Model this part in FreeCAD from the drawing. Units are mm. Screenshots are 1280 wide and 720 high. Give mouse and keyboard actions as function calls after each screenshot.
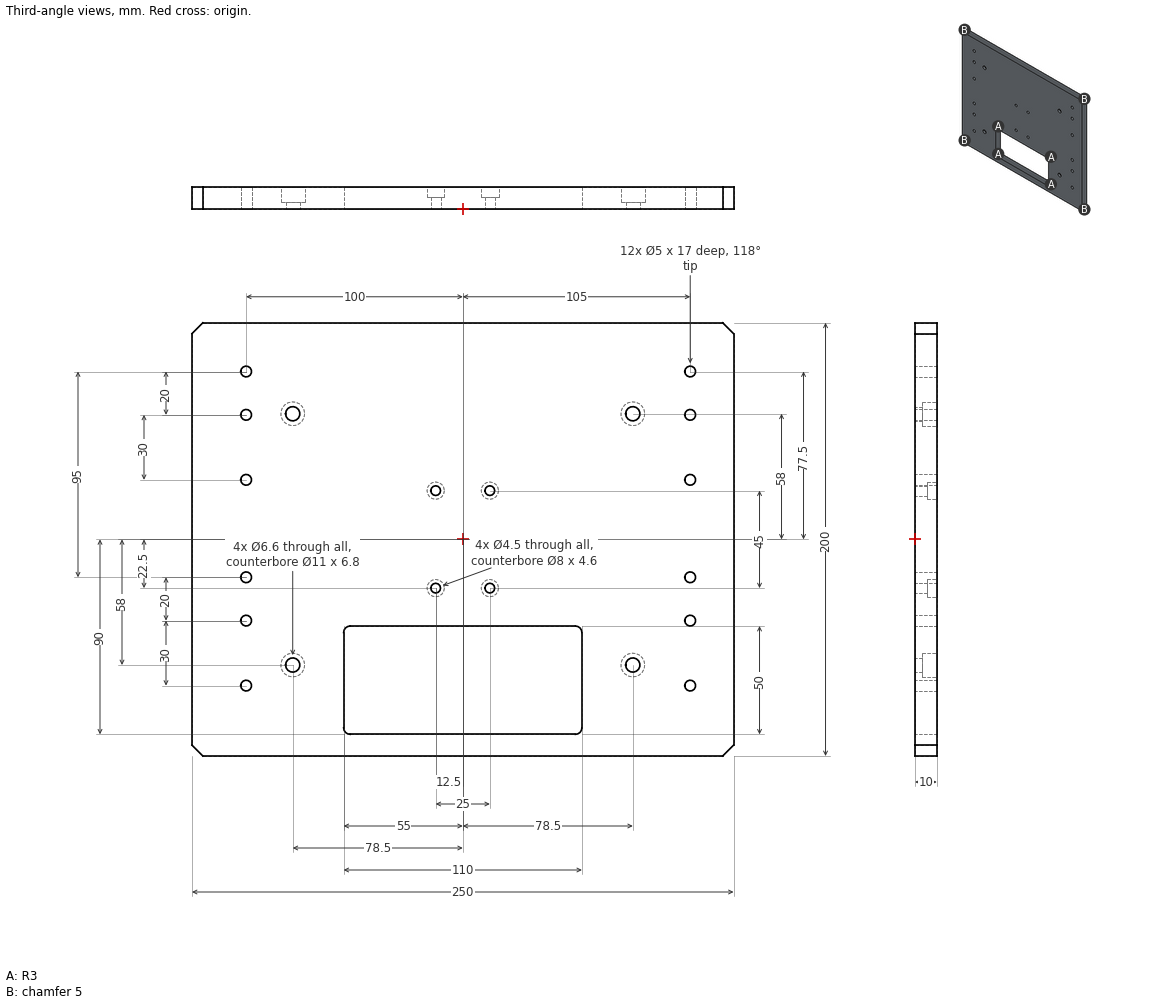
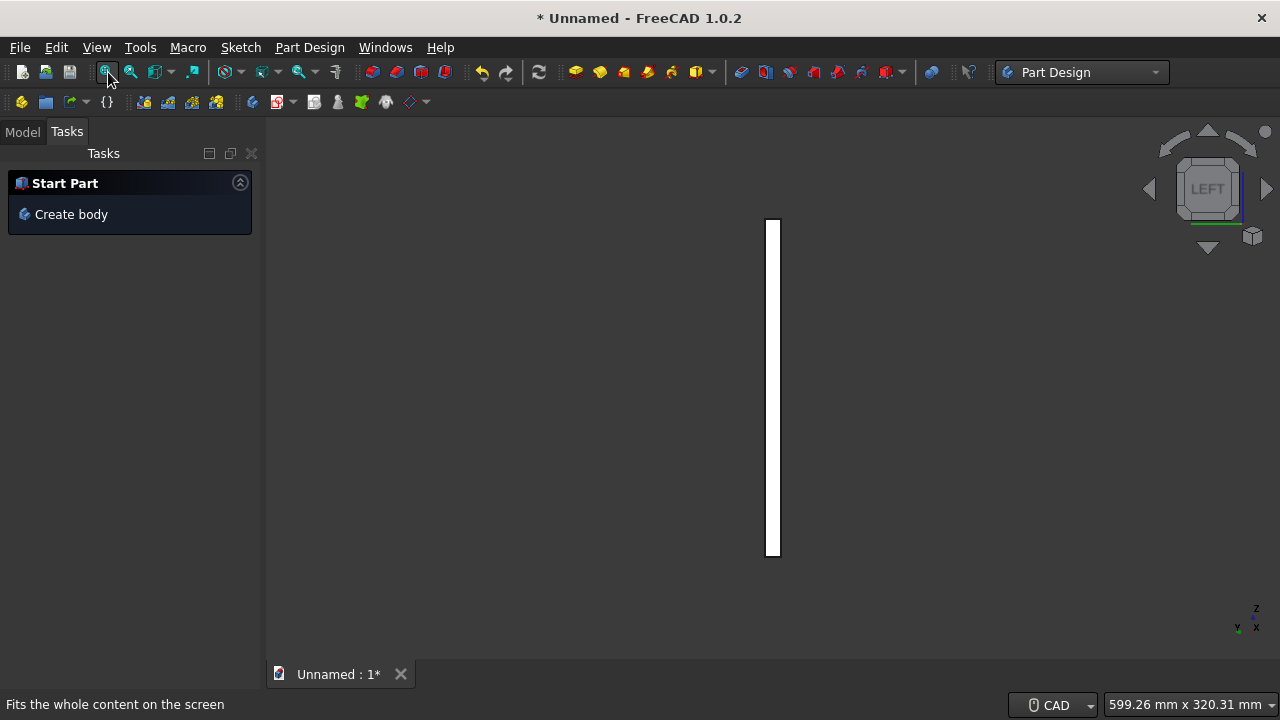
scroll(773, 455, up, 5)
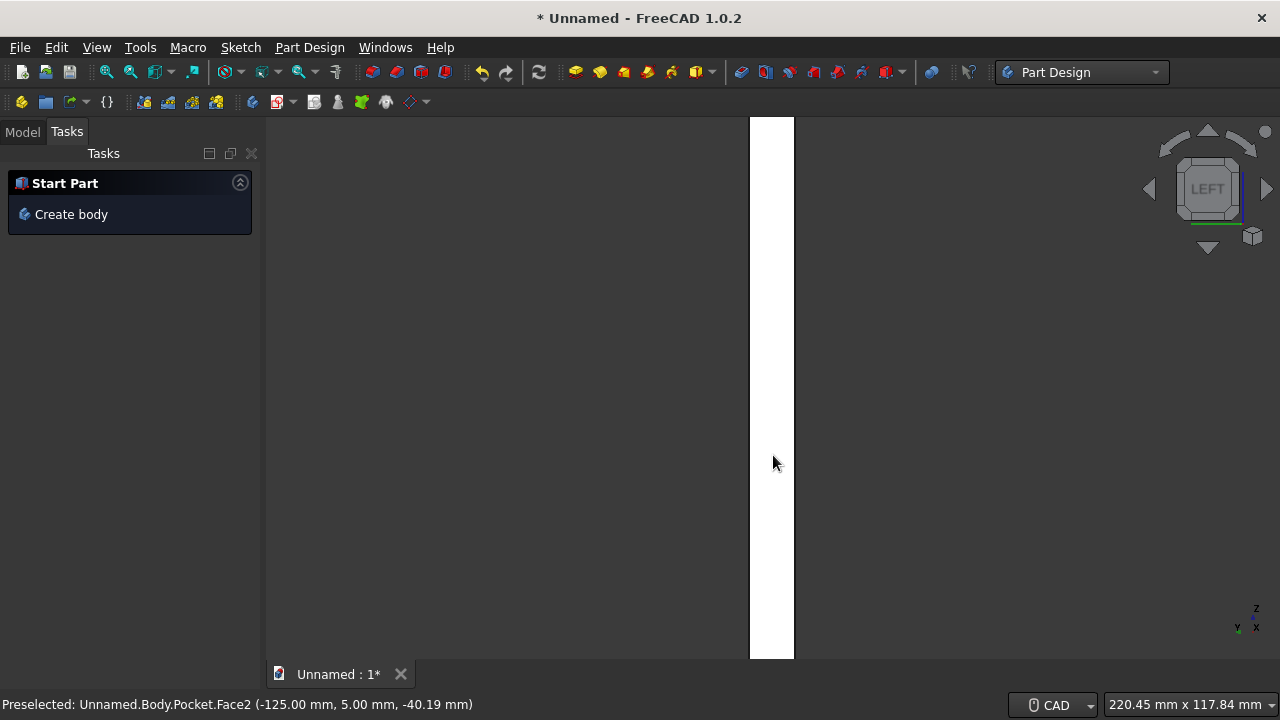
click(108, 72)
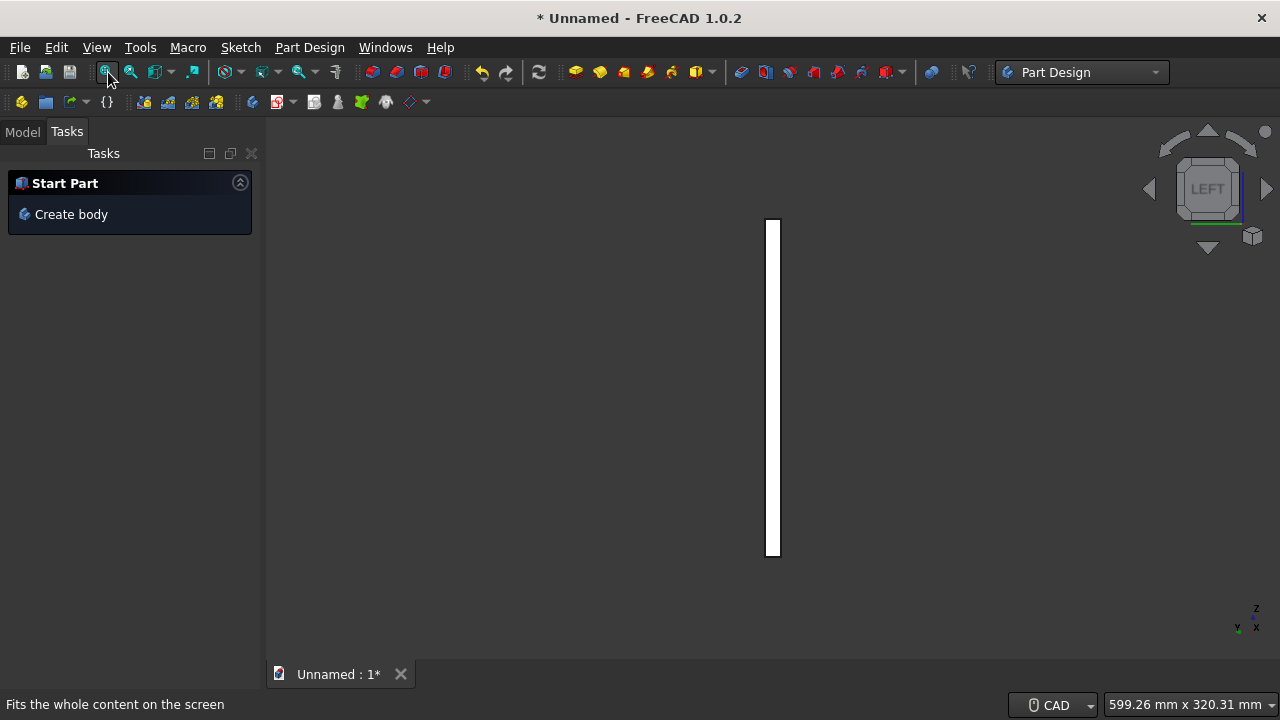
key(v)
key(3)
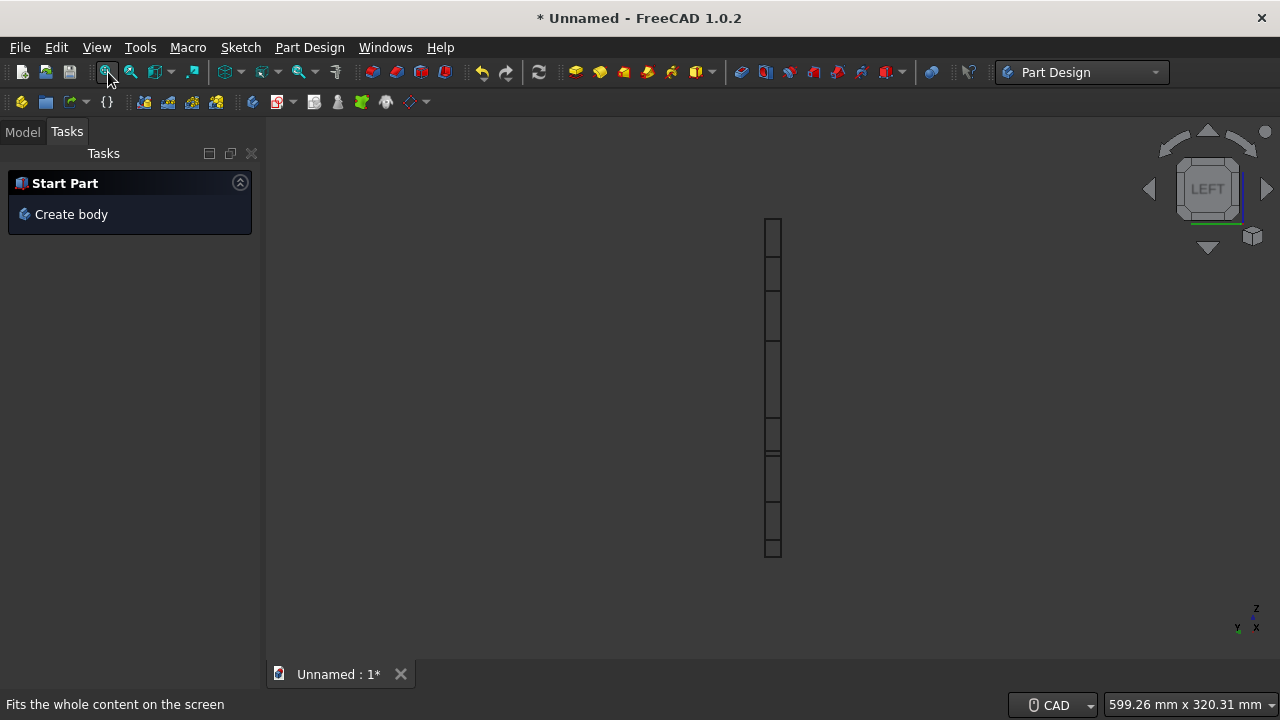
key(0)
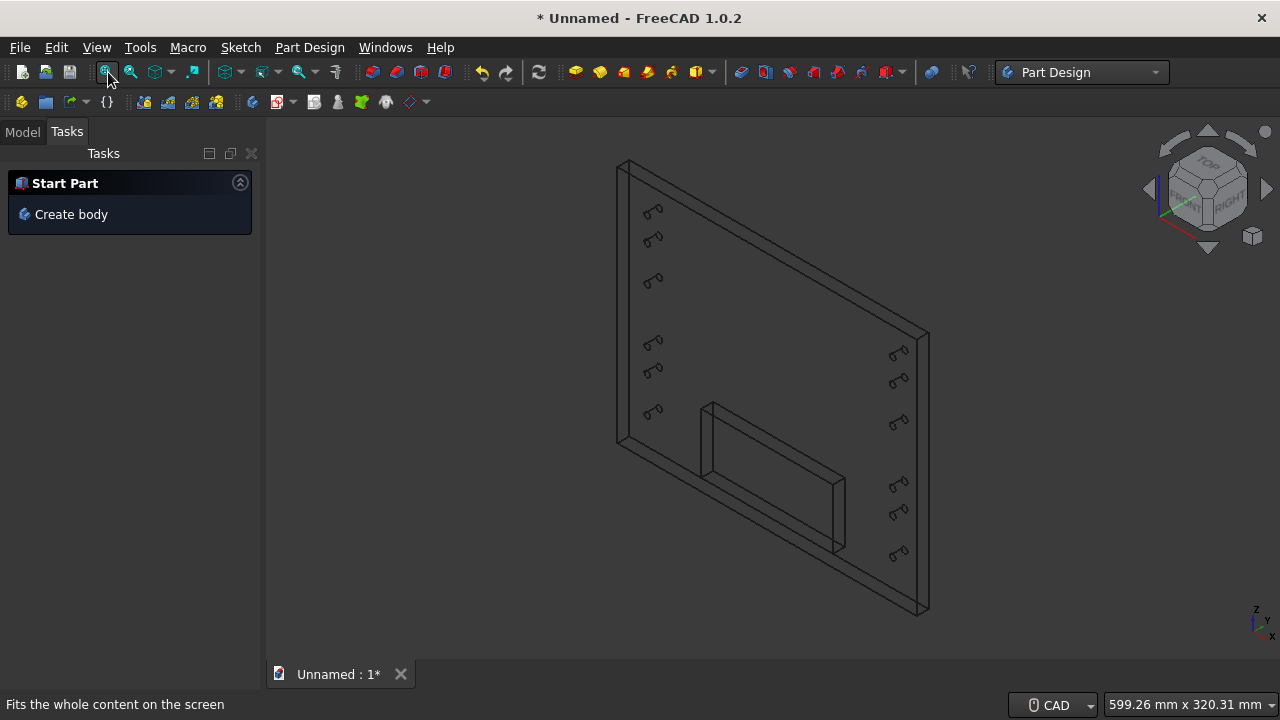
click(708, 404)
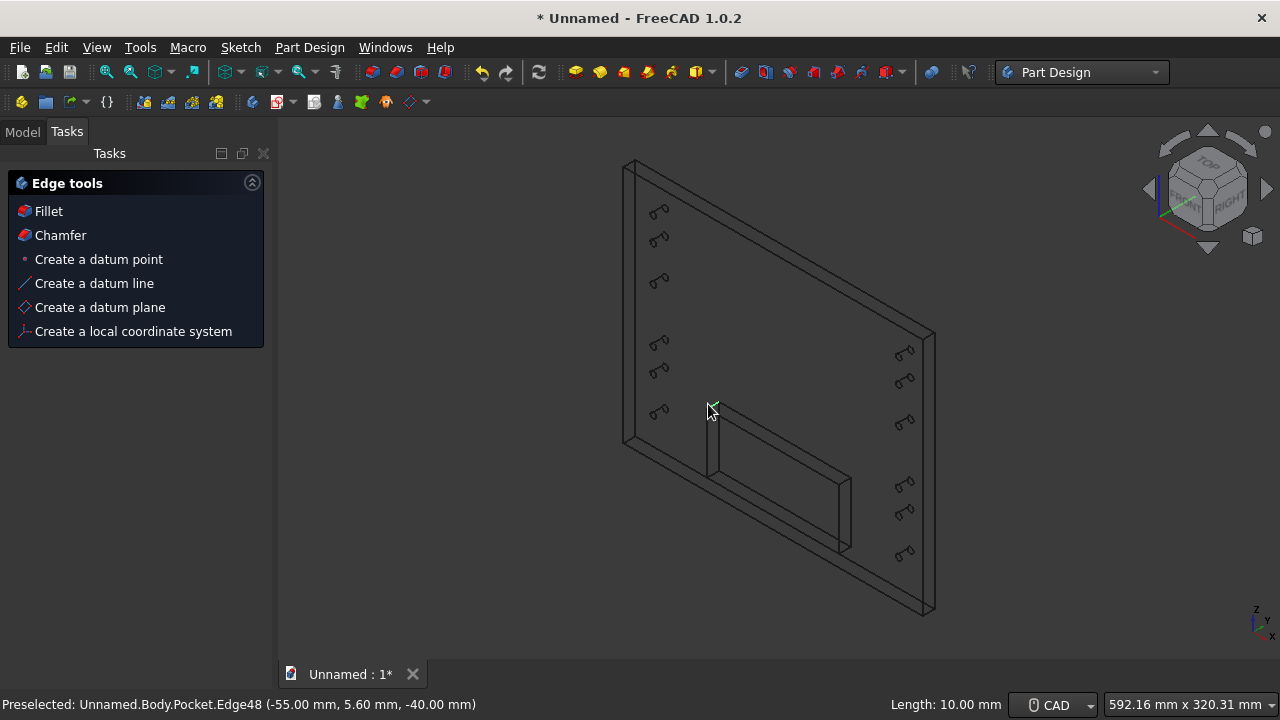
click(714, 473, ctrl)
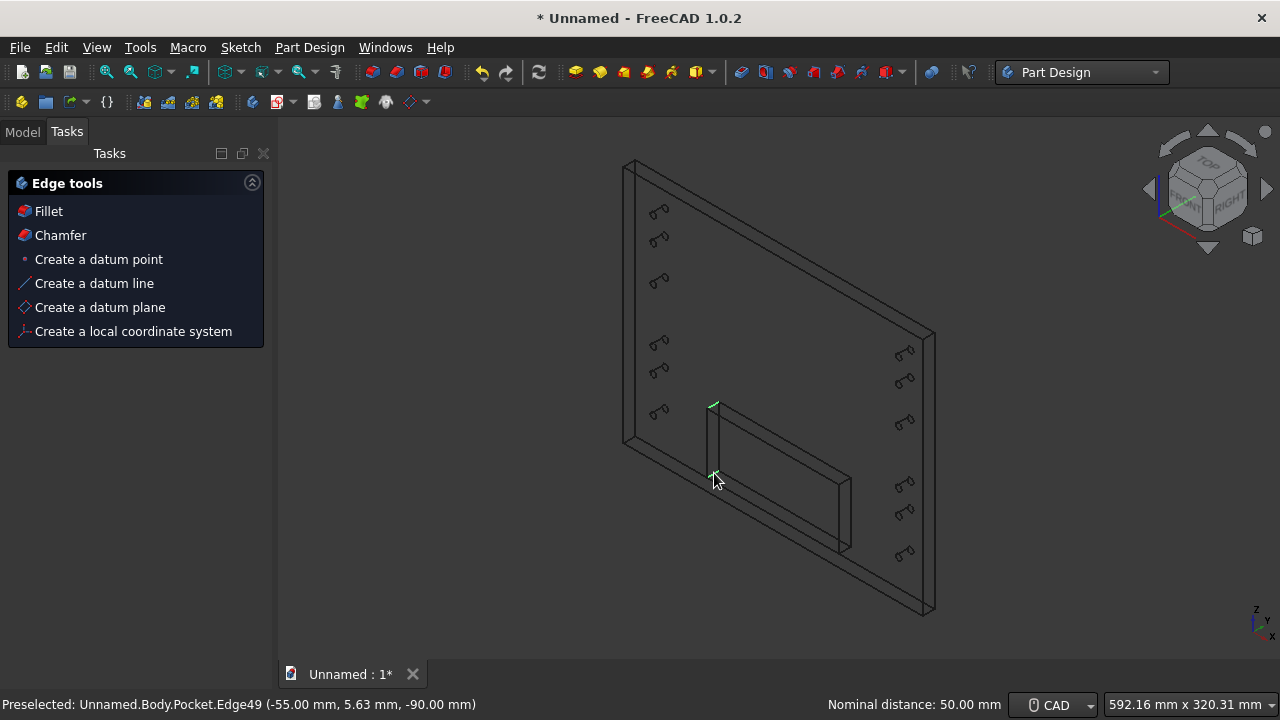
click(845, 549, ctrl)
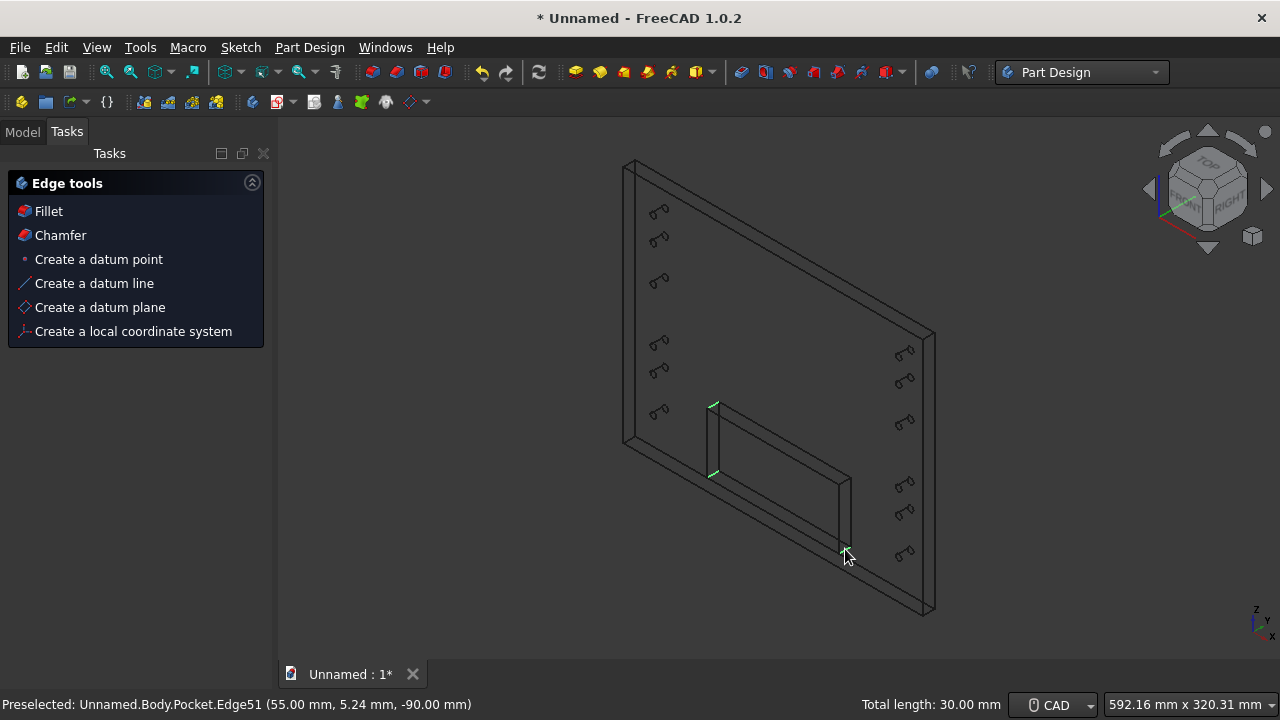
click(845, 480, ctrl)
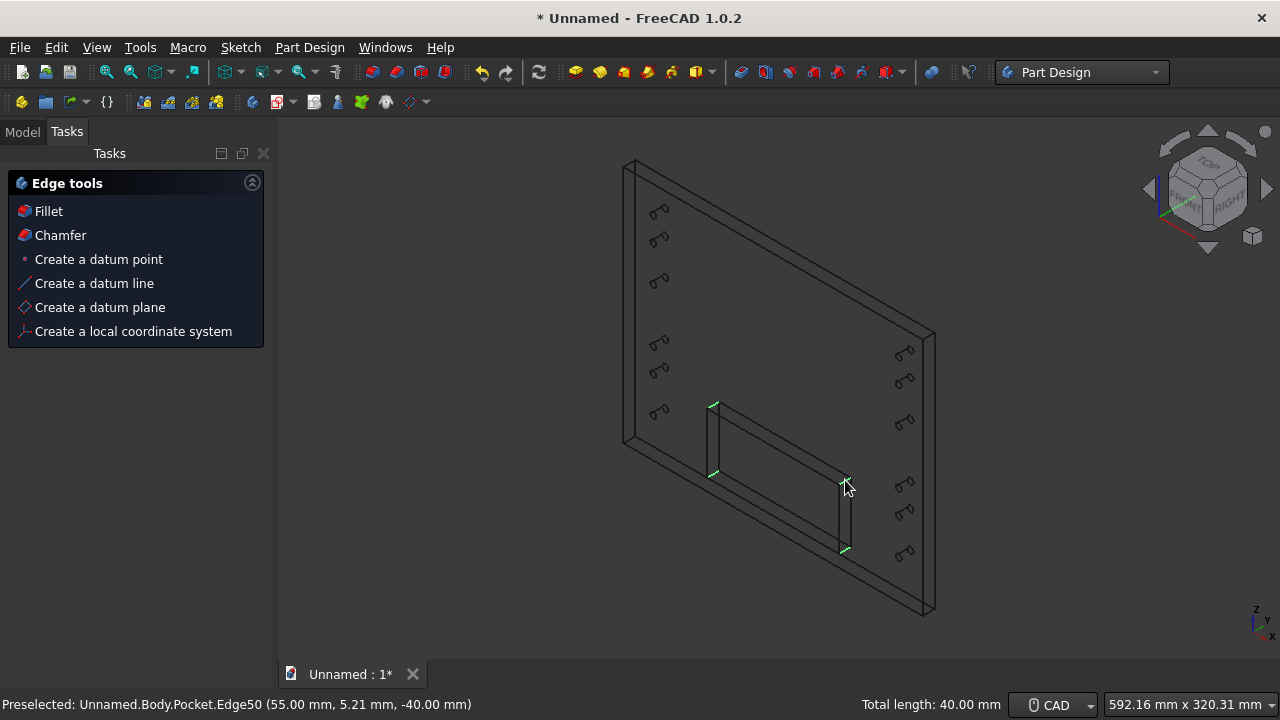
key(v)
key(1)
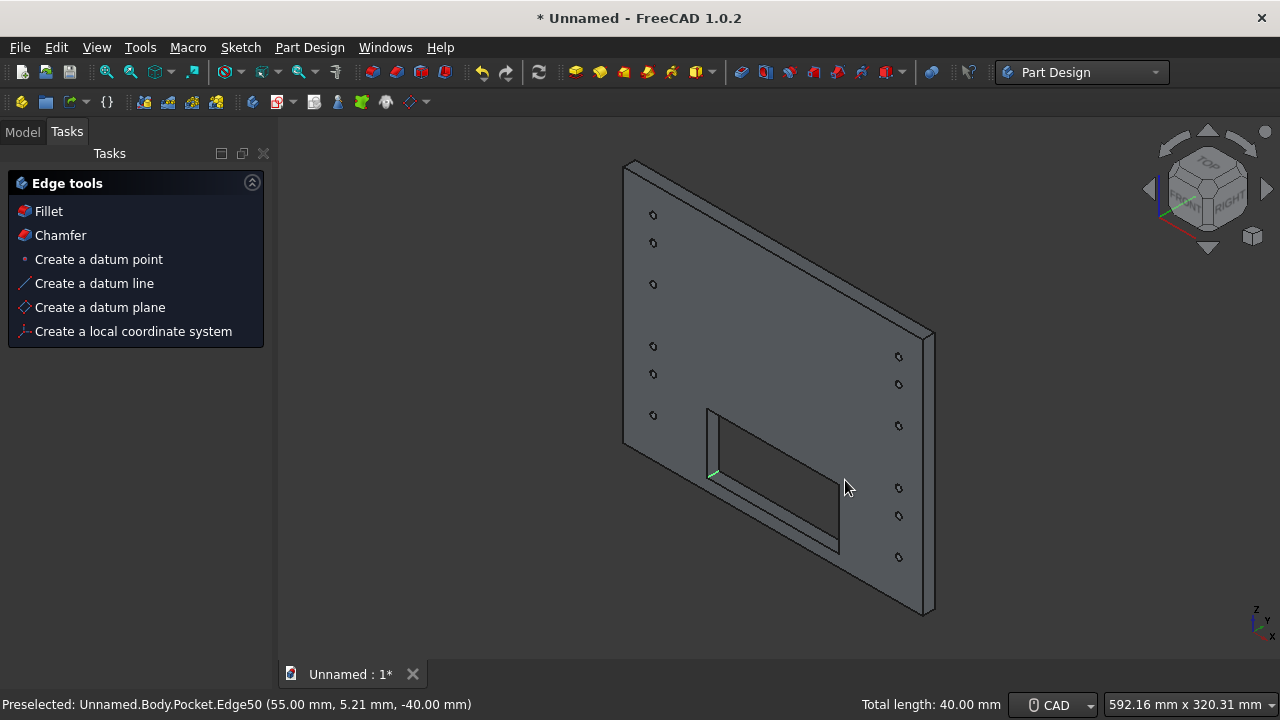
click(374, 72)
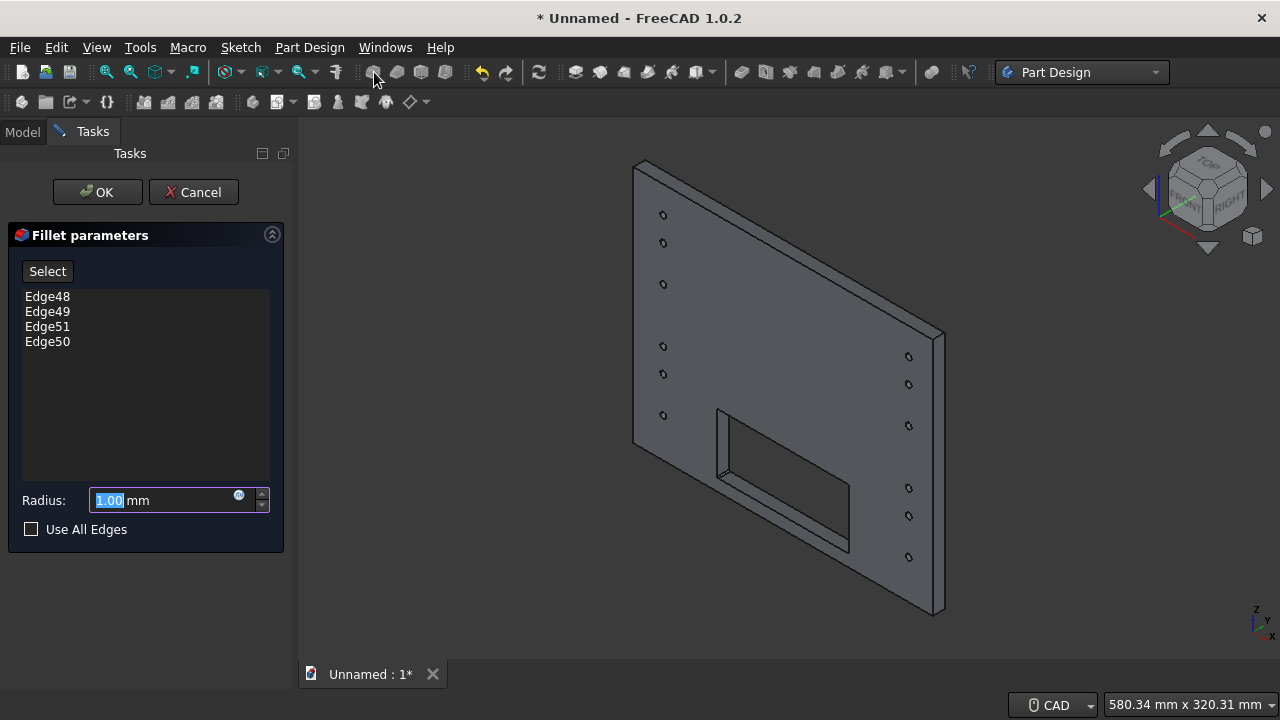
text(3)
key(Tab)